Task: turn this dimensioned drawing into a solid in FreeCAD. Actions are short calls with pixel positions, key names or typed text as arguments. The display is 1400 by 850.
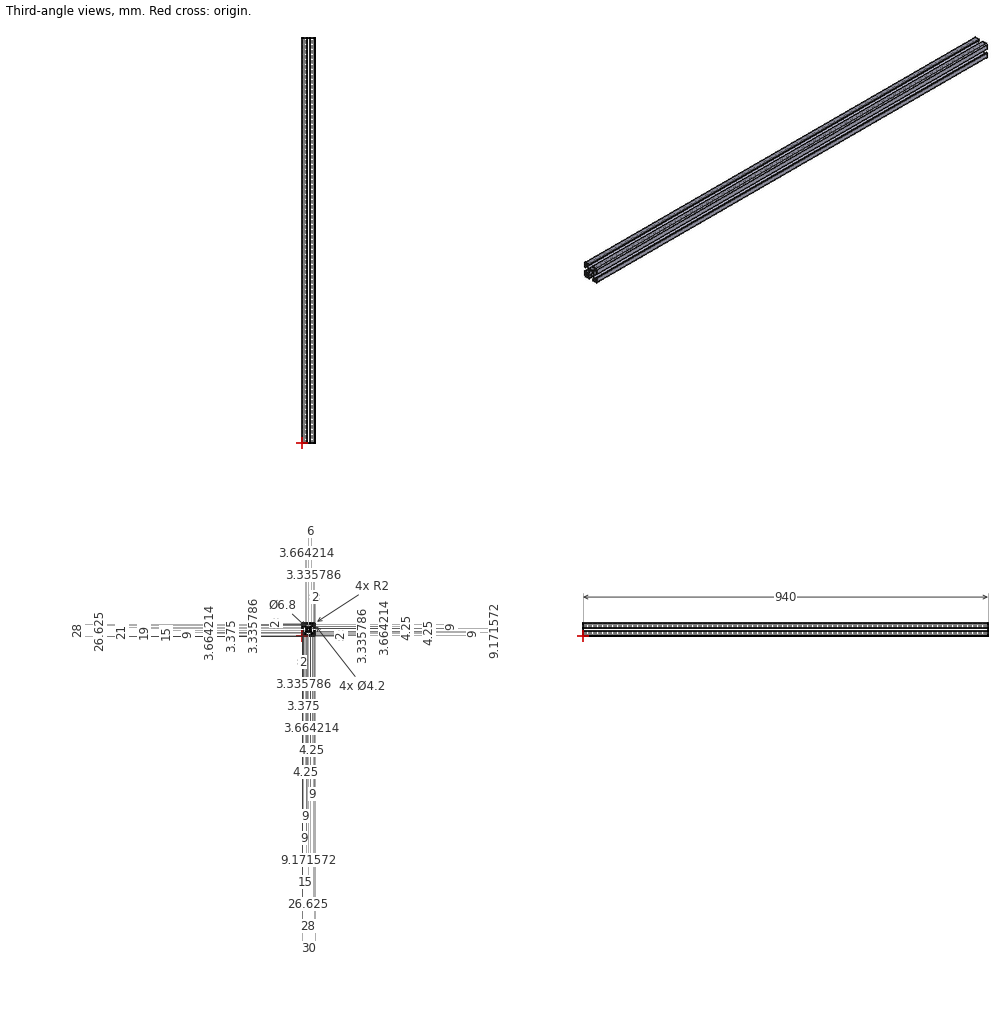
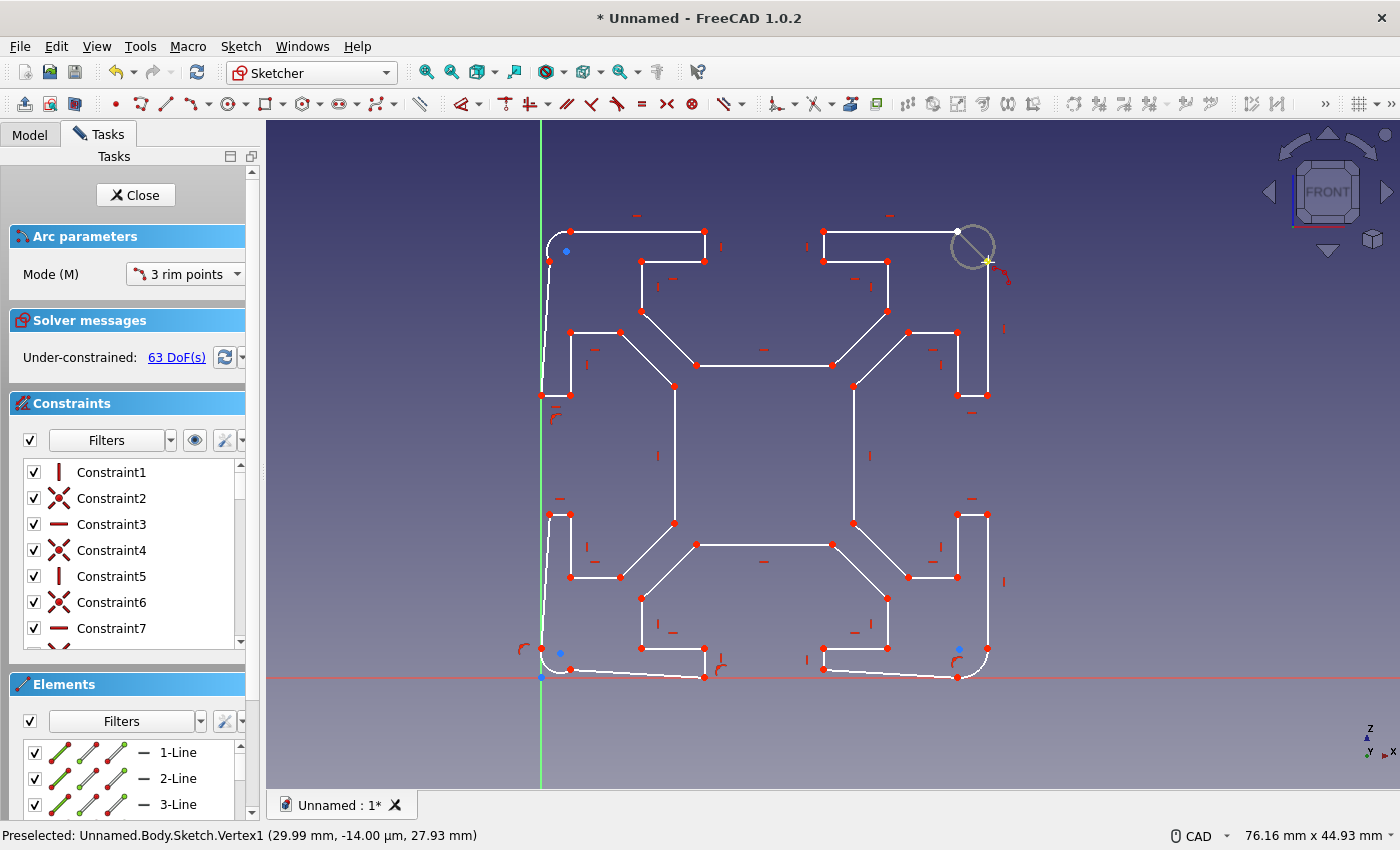
scroll(979, 240, up, 3)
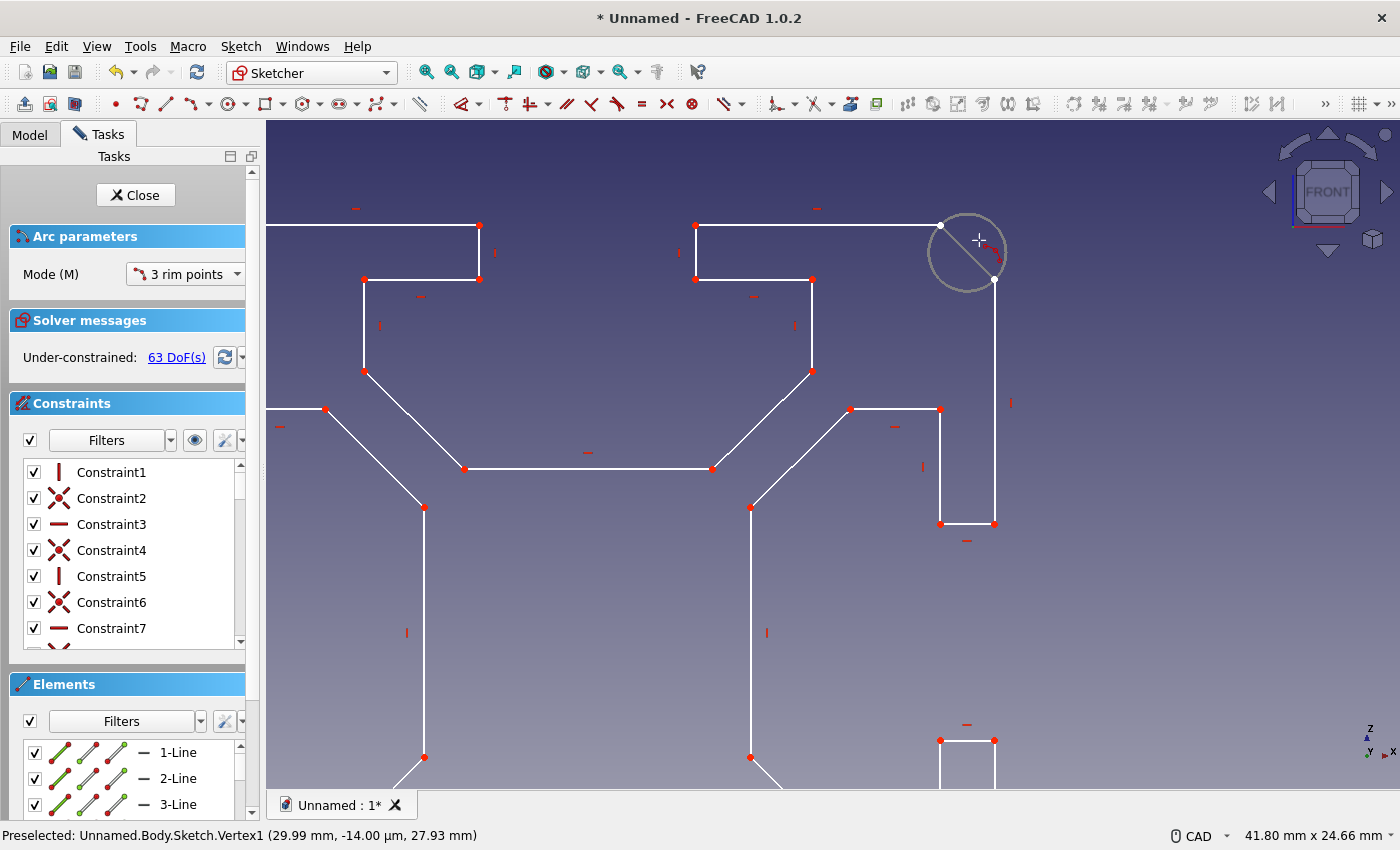
click(979, 240)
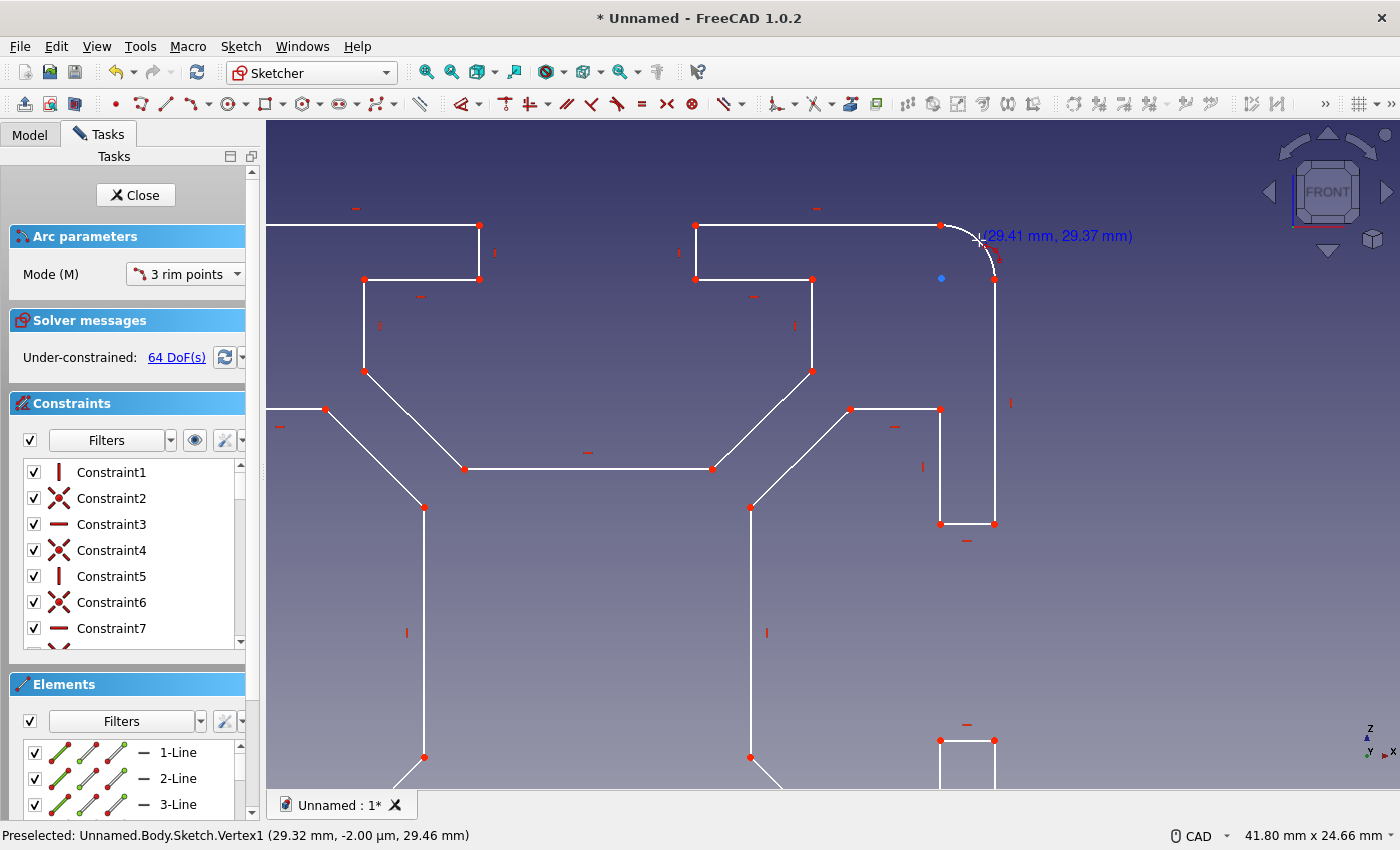
key(g)
key(c)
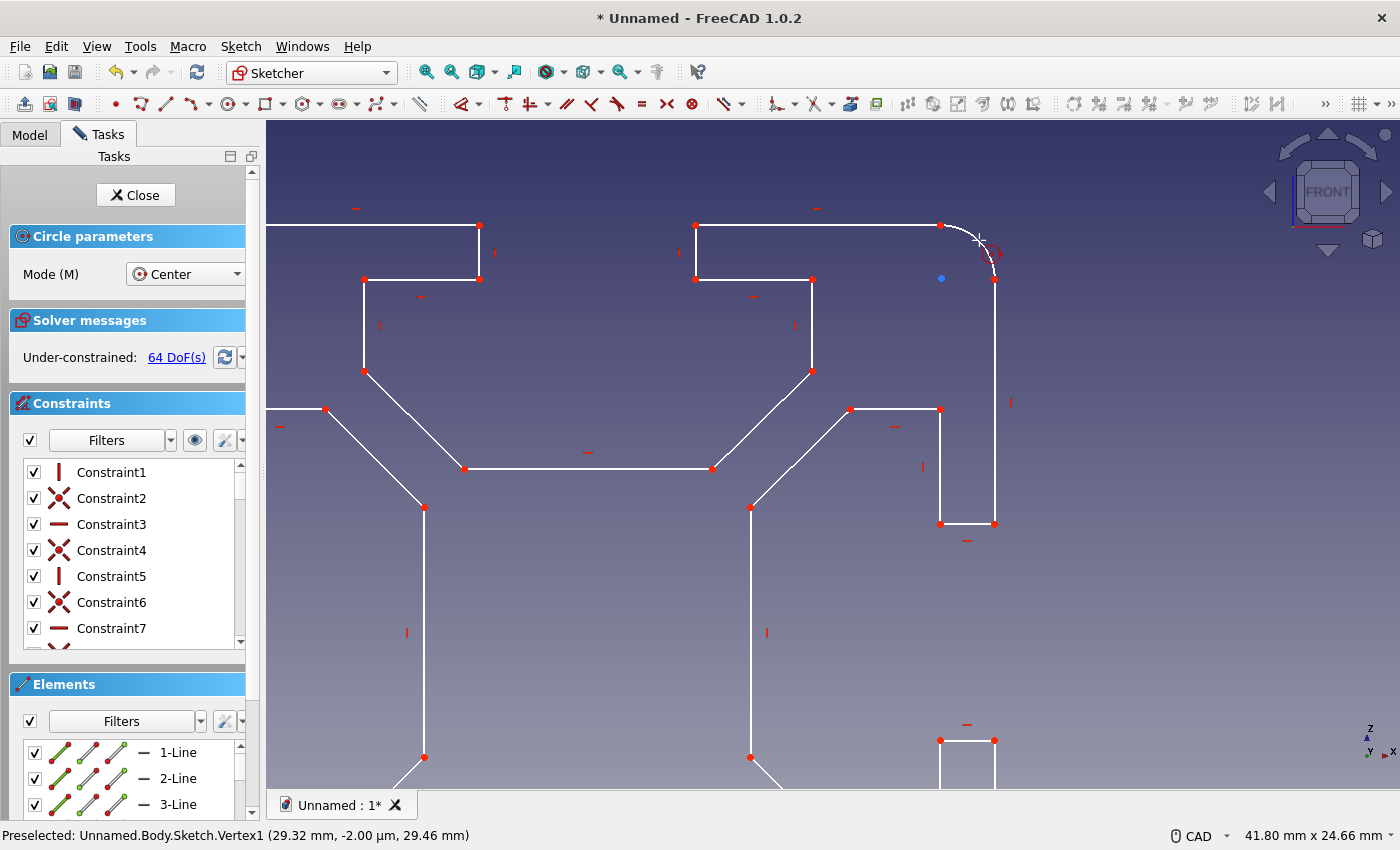
click(903, 315)
click(863, 275)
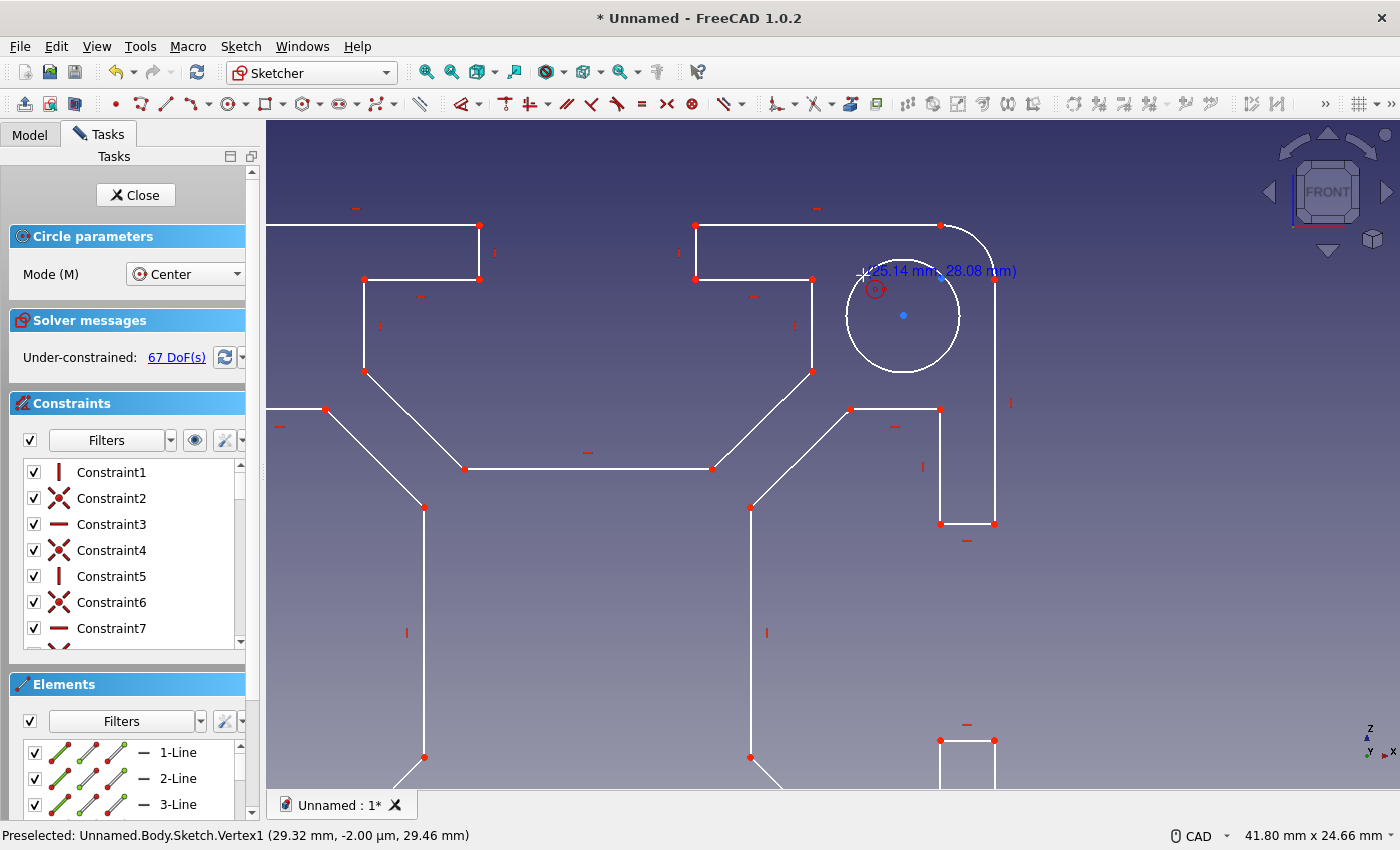
scroll(979, 240, down, 3)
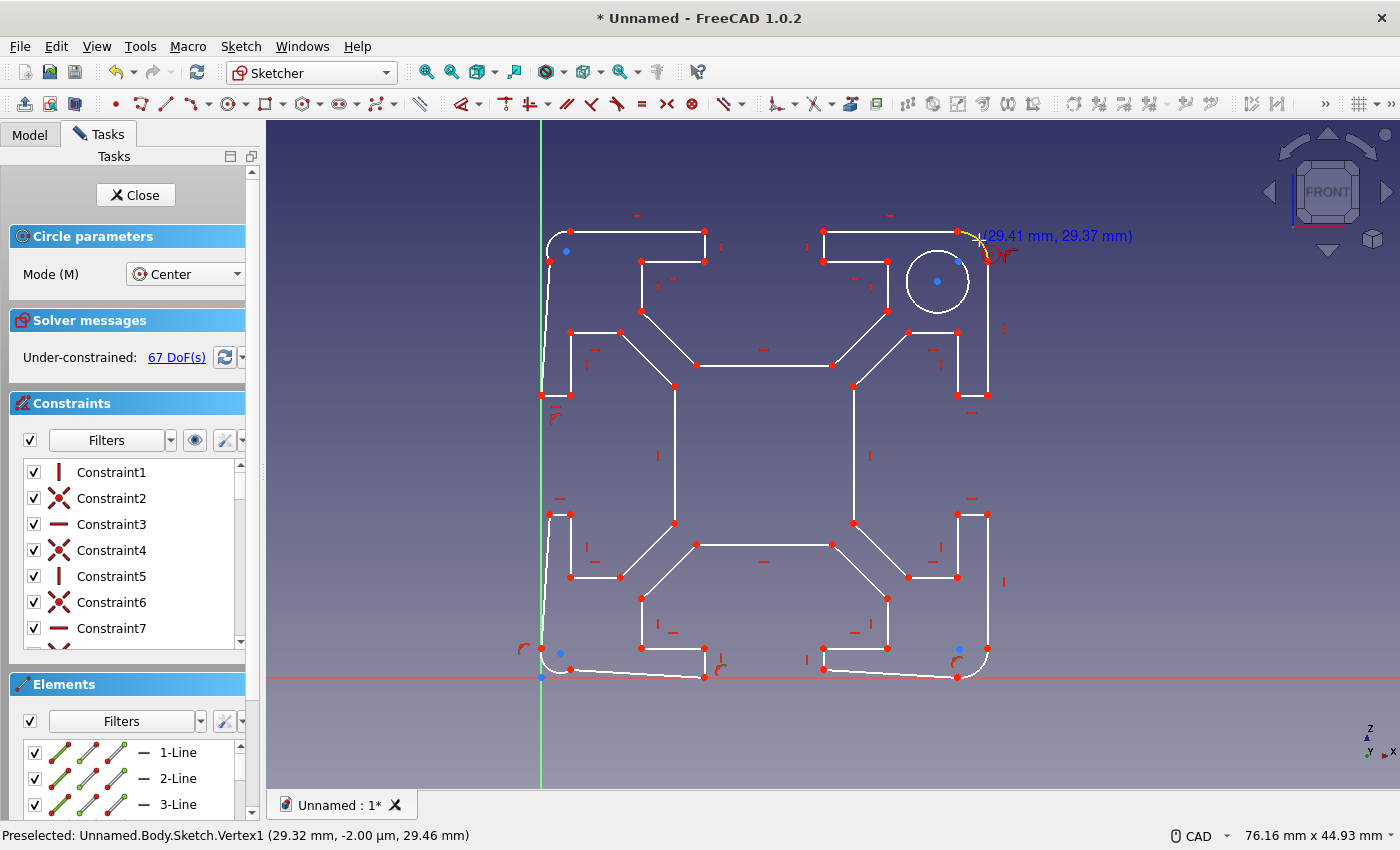
click(592, 281)
click(614, 259)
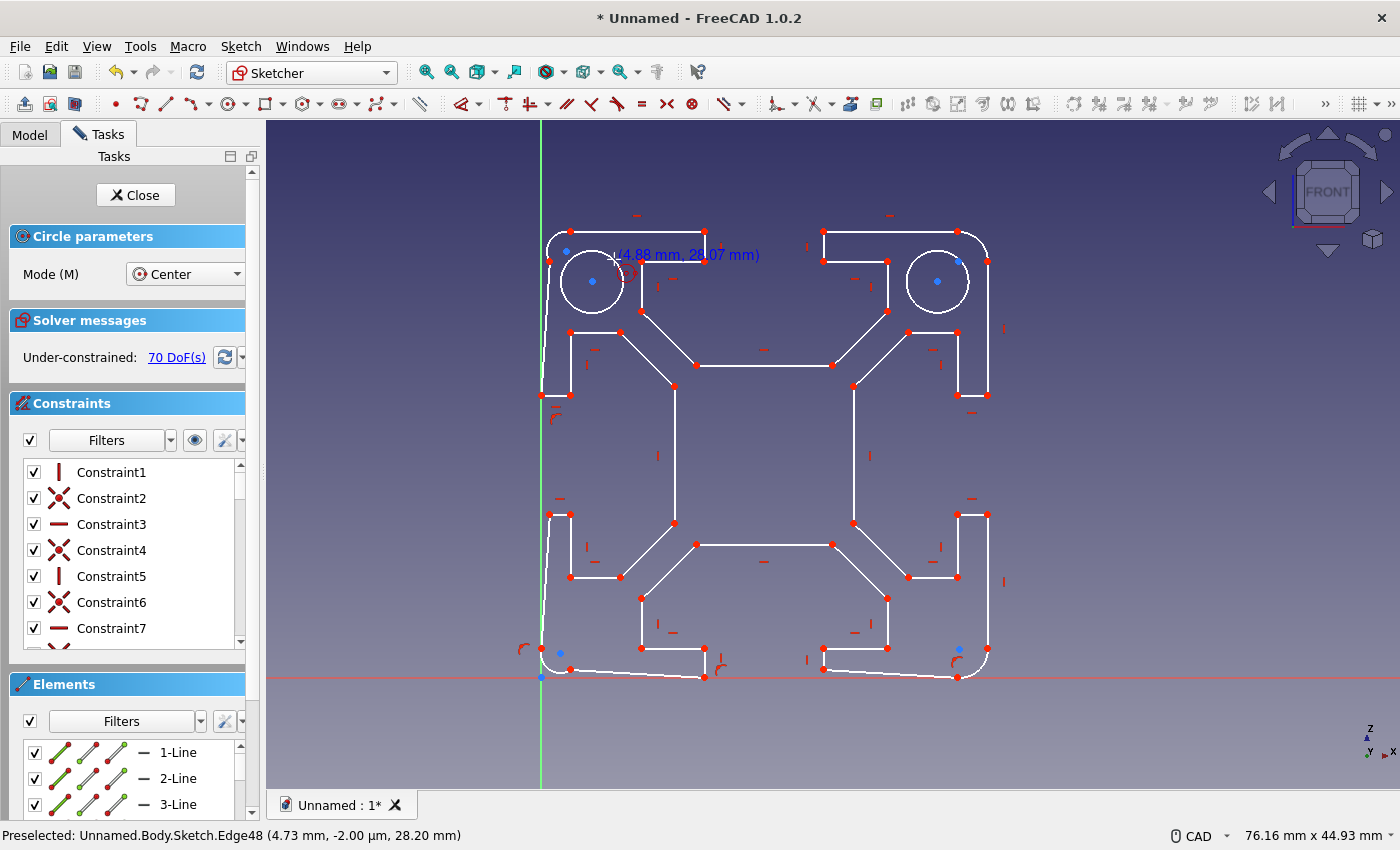
click(938, 628)
click(960, 606)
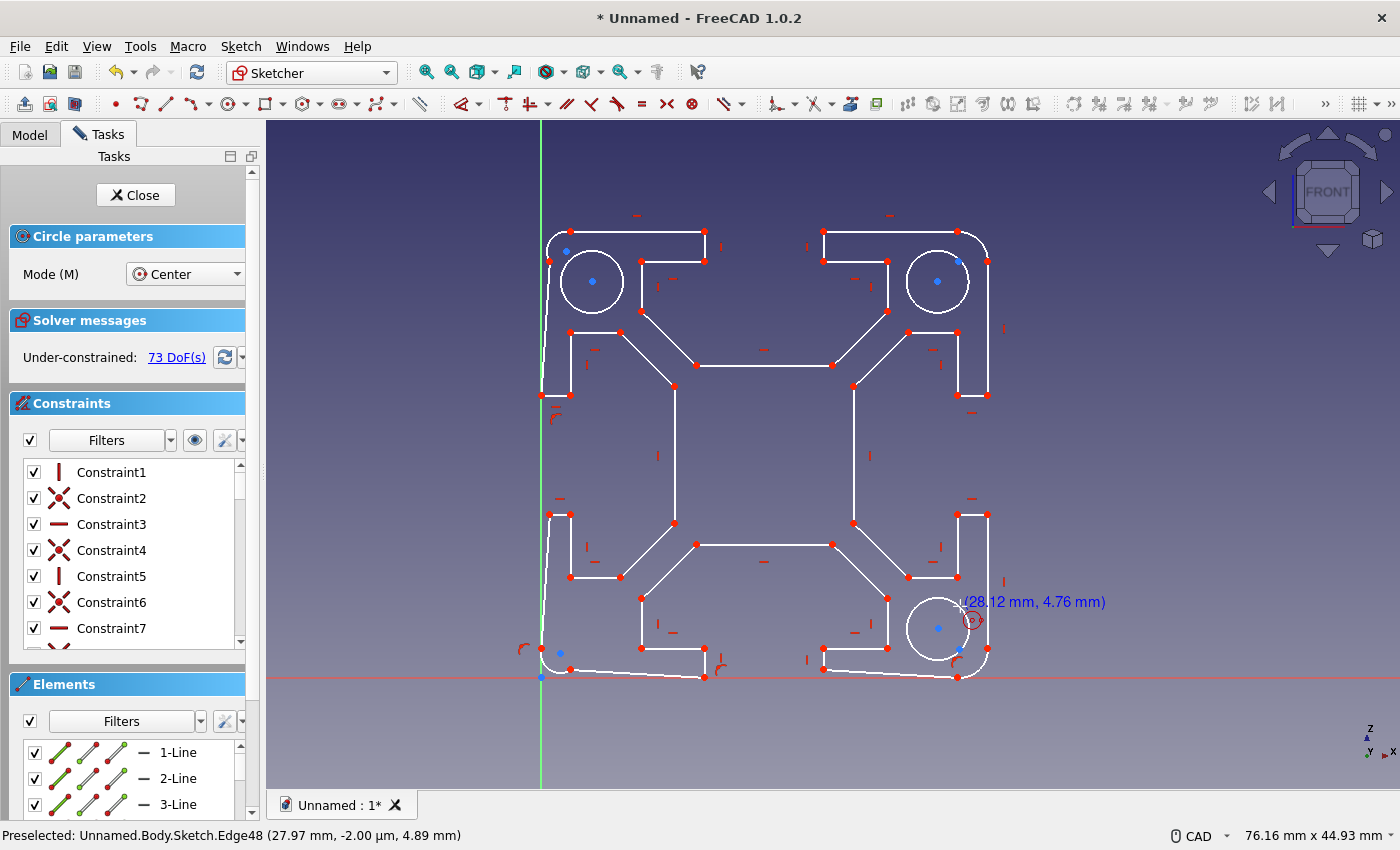
click(765, 455)
click(800, 419)